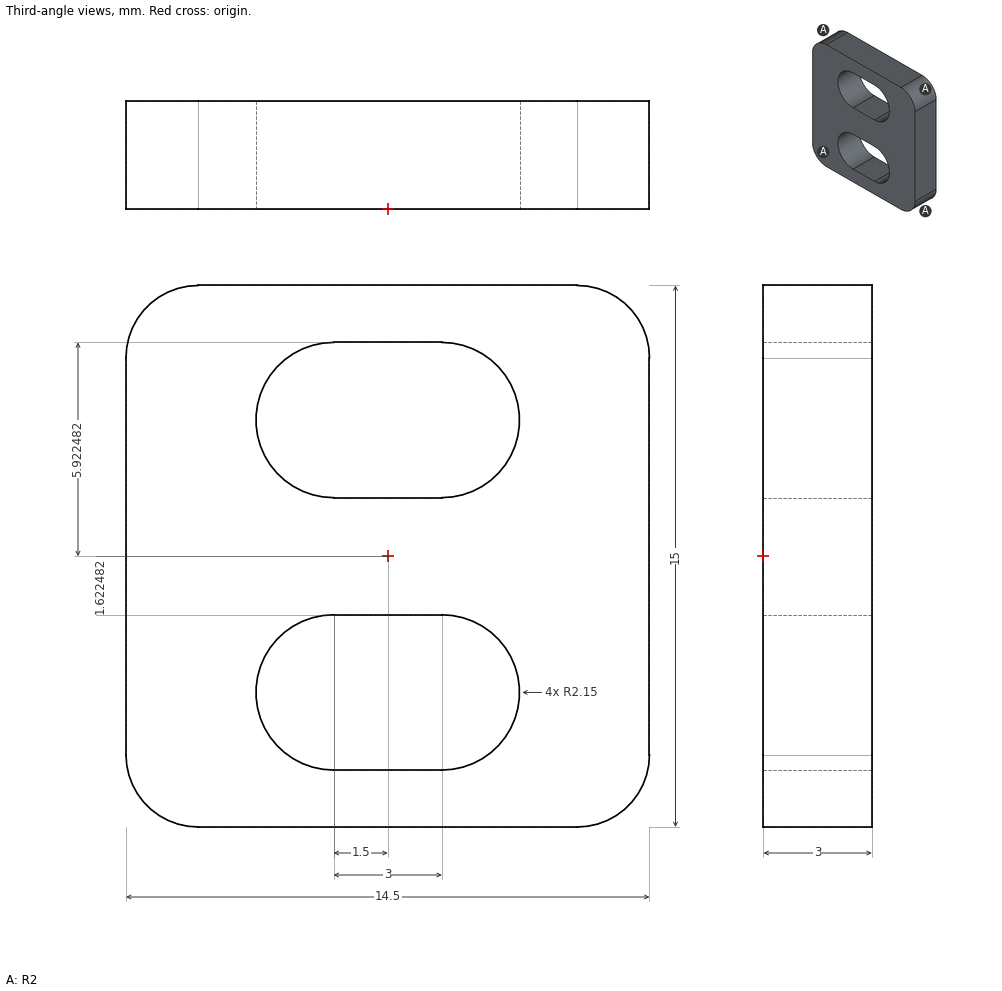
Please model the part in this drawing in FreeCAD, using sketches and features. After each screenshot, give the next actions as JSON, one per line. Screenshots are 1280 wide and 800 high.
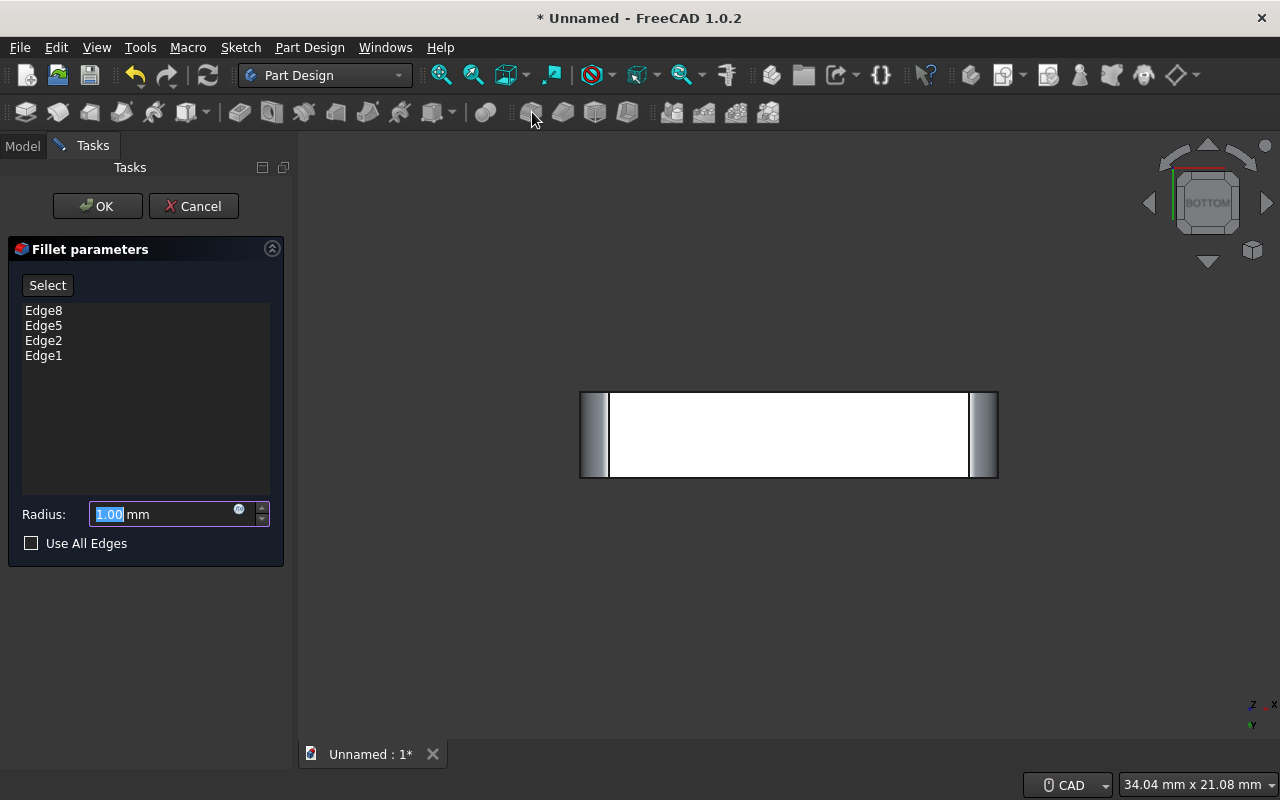
{"action": "type", "text": "2"}
{"action": "key", "text": "Tab"}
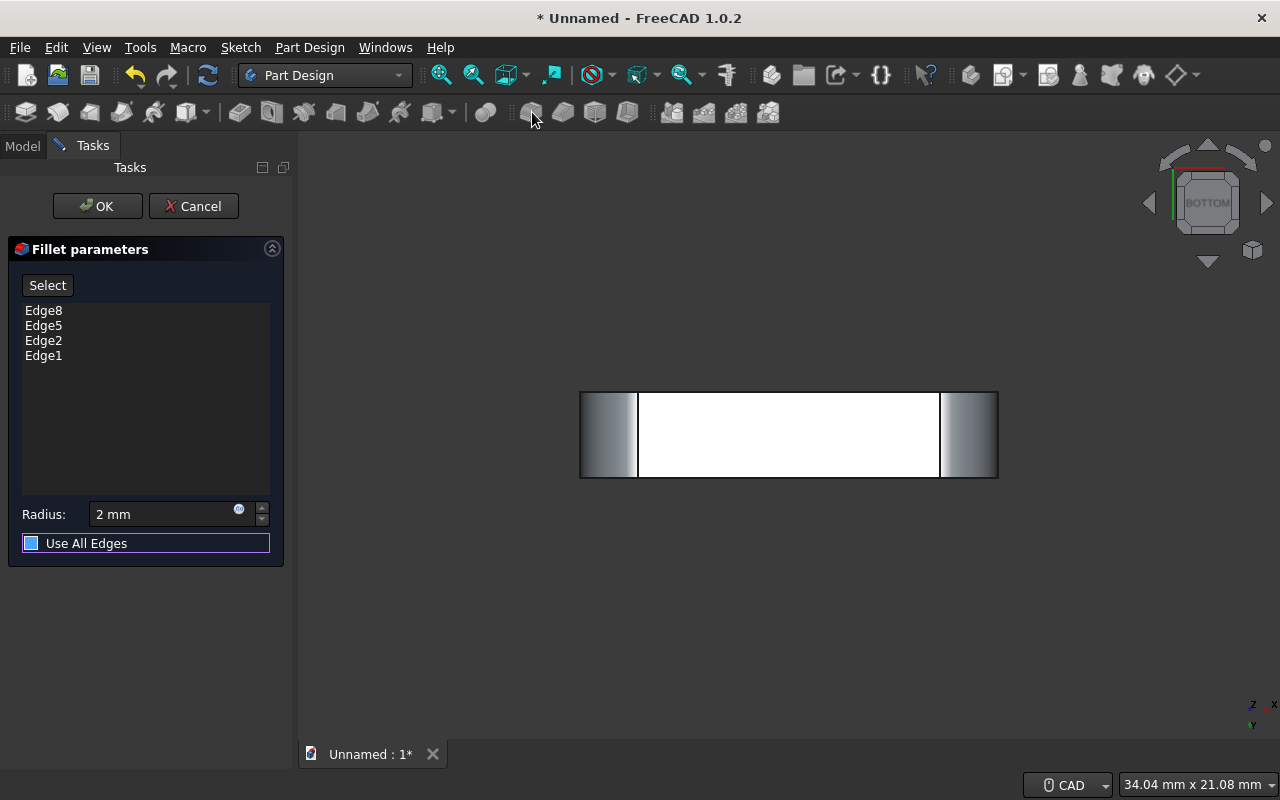
{"action": "left_click", "coordinate": [98, 206]}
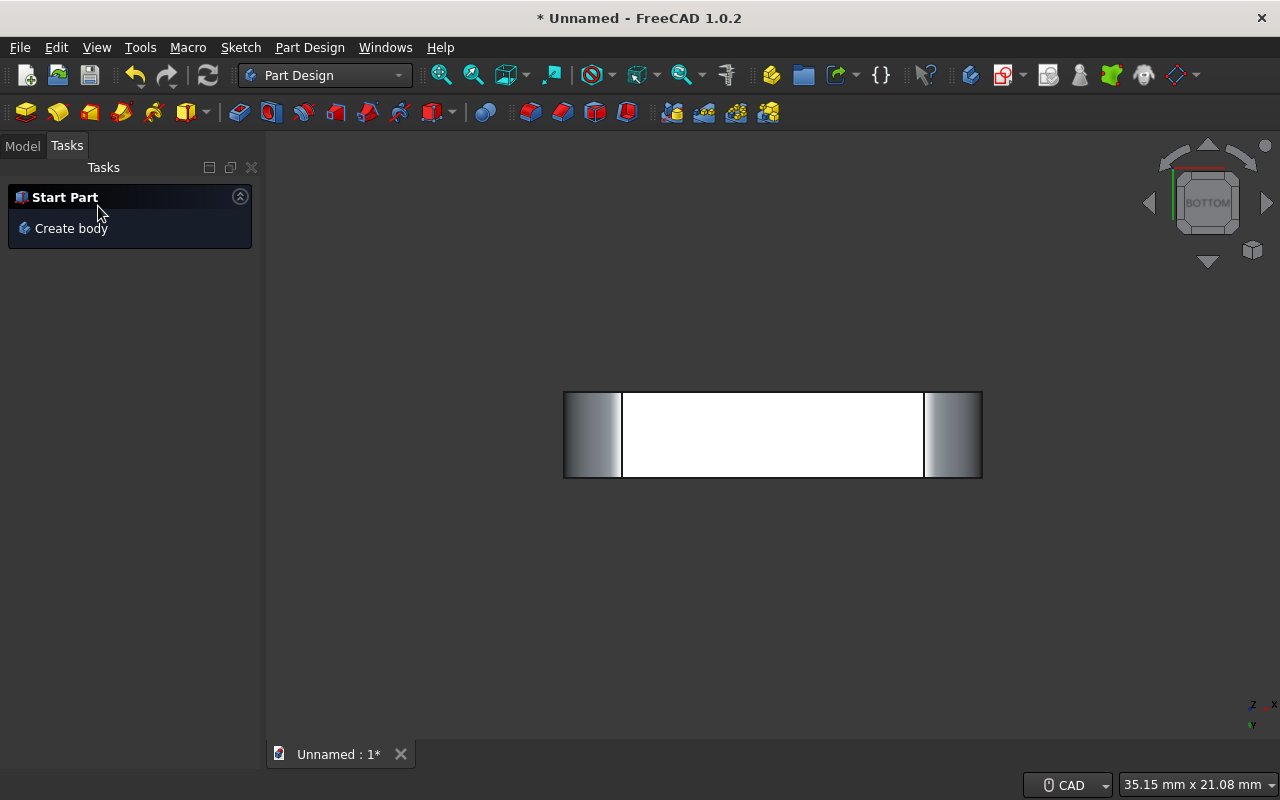
{"action": "key", "text": "0"}